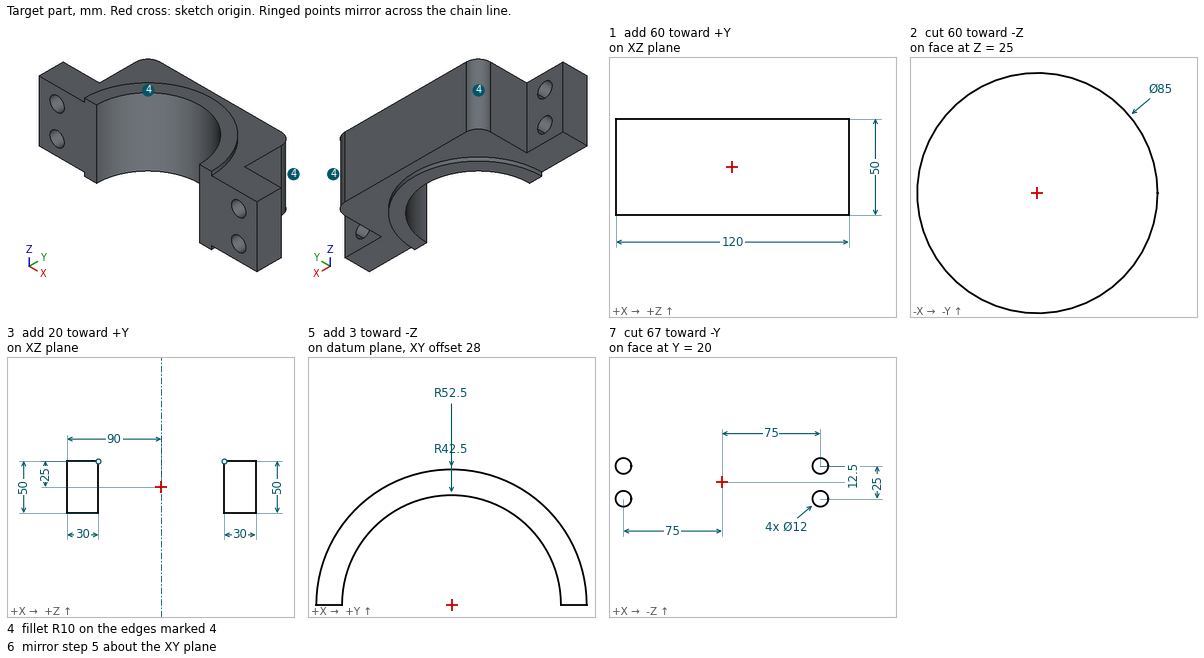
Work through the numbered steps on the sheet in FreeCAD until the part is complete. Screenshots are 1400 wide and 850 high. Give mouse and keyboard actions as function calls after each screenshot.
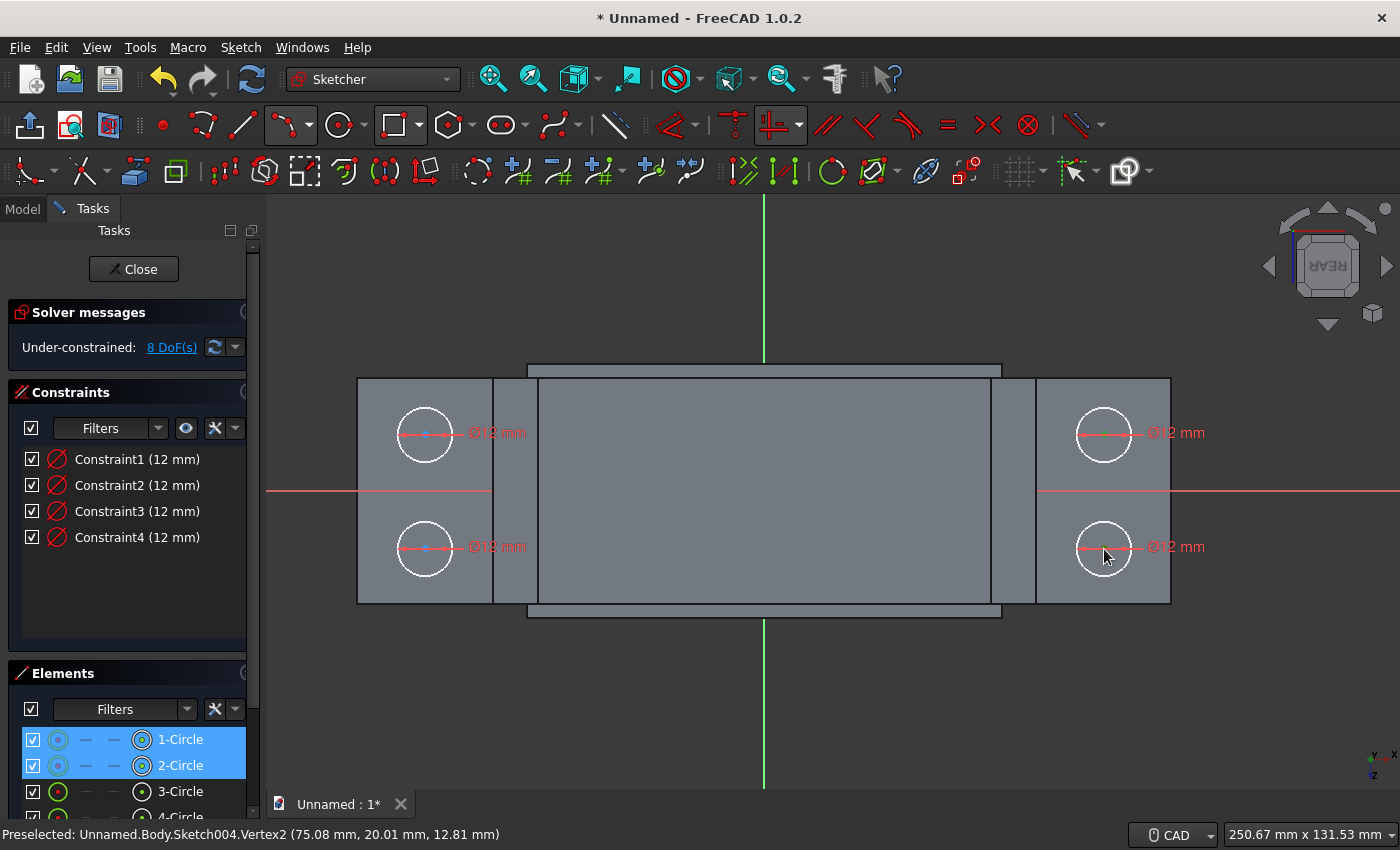
click(802, 126)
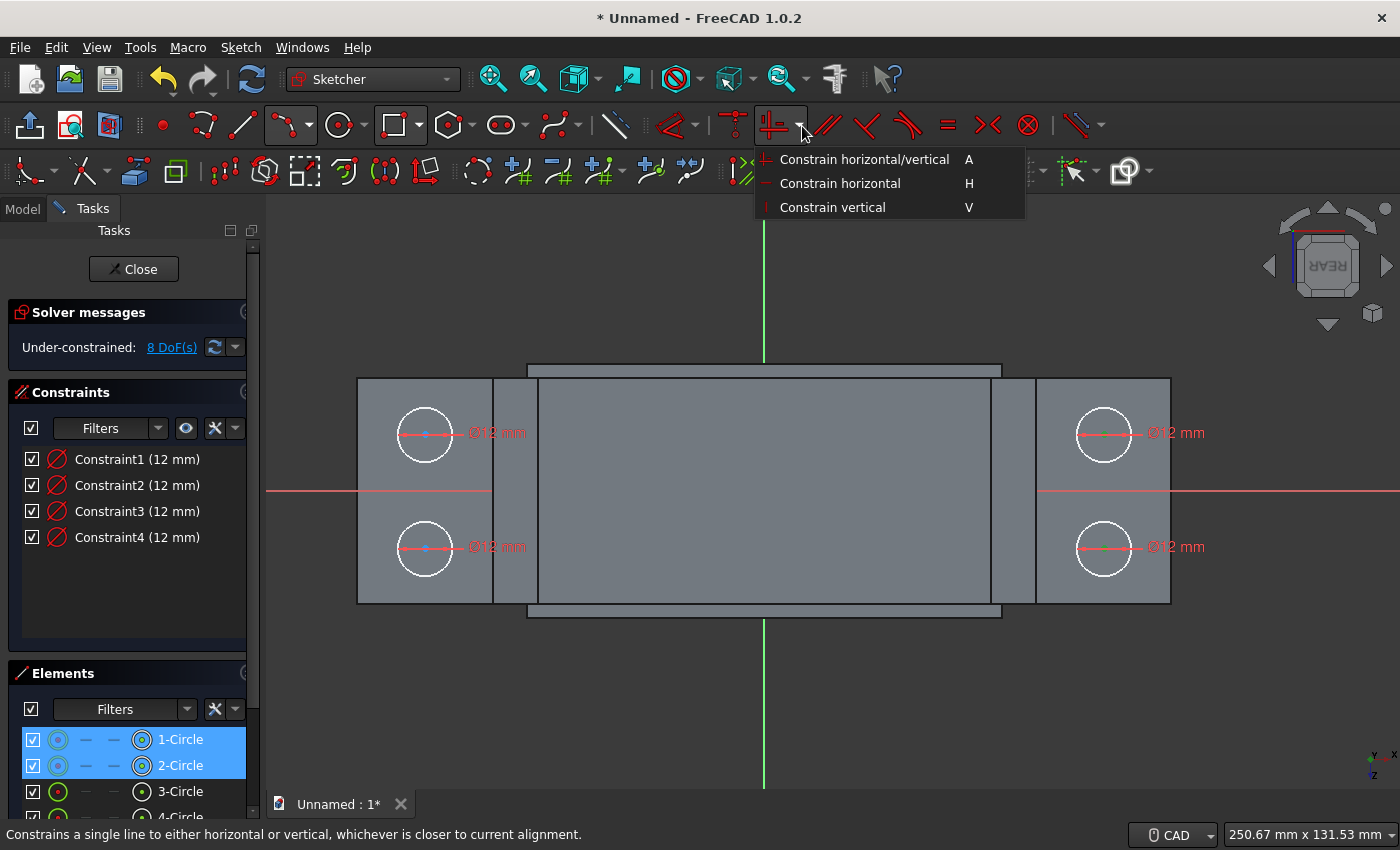
click(890, 207)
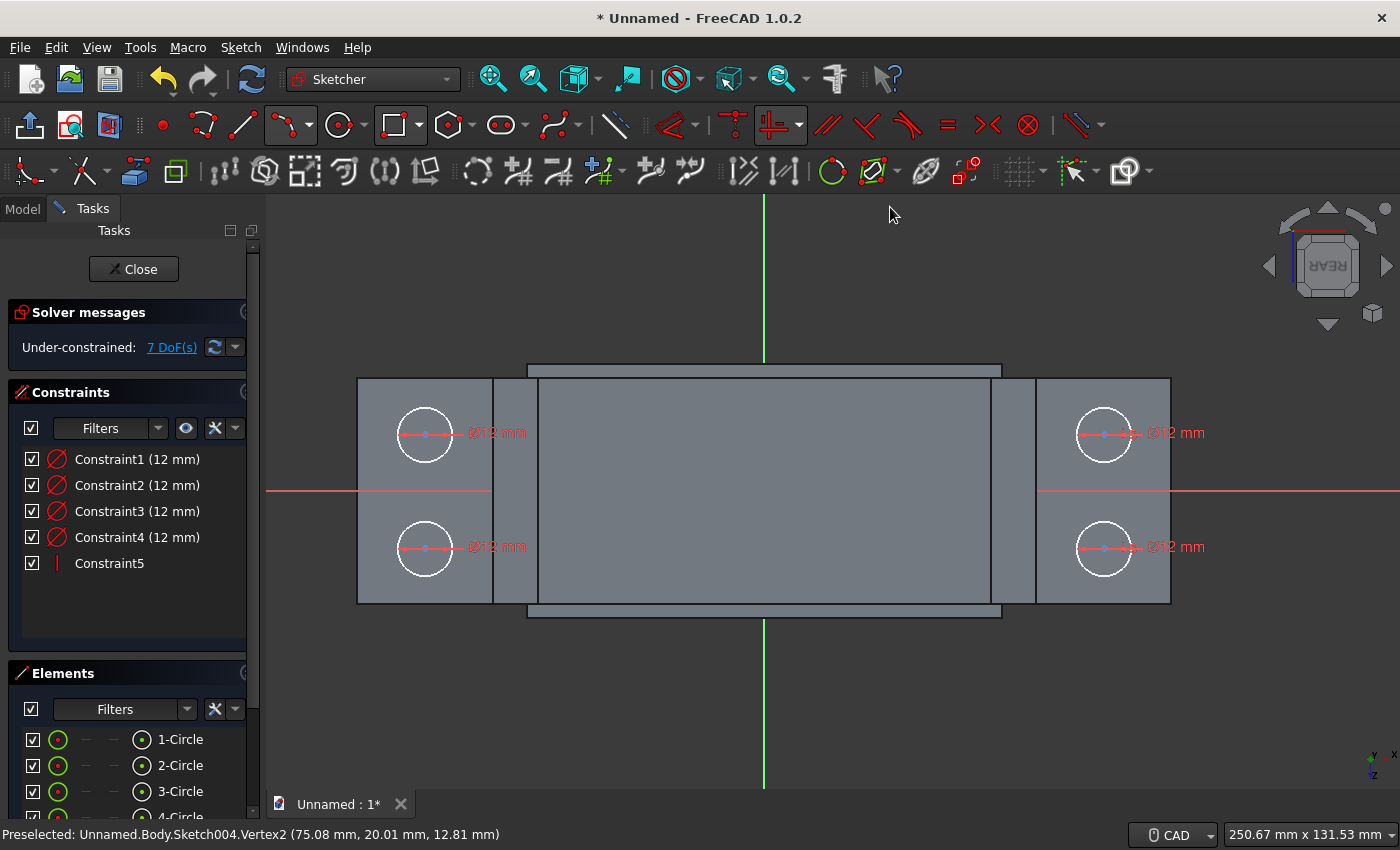
click(1104, 549)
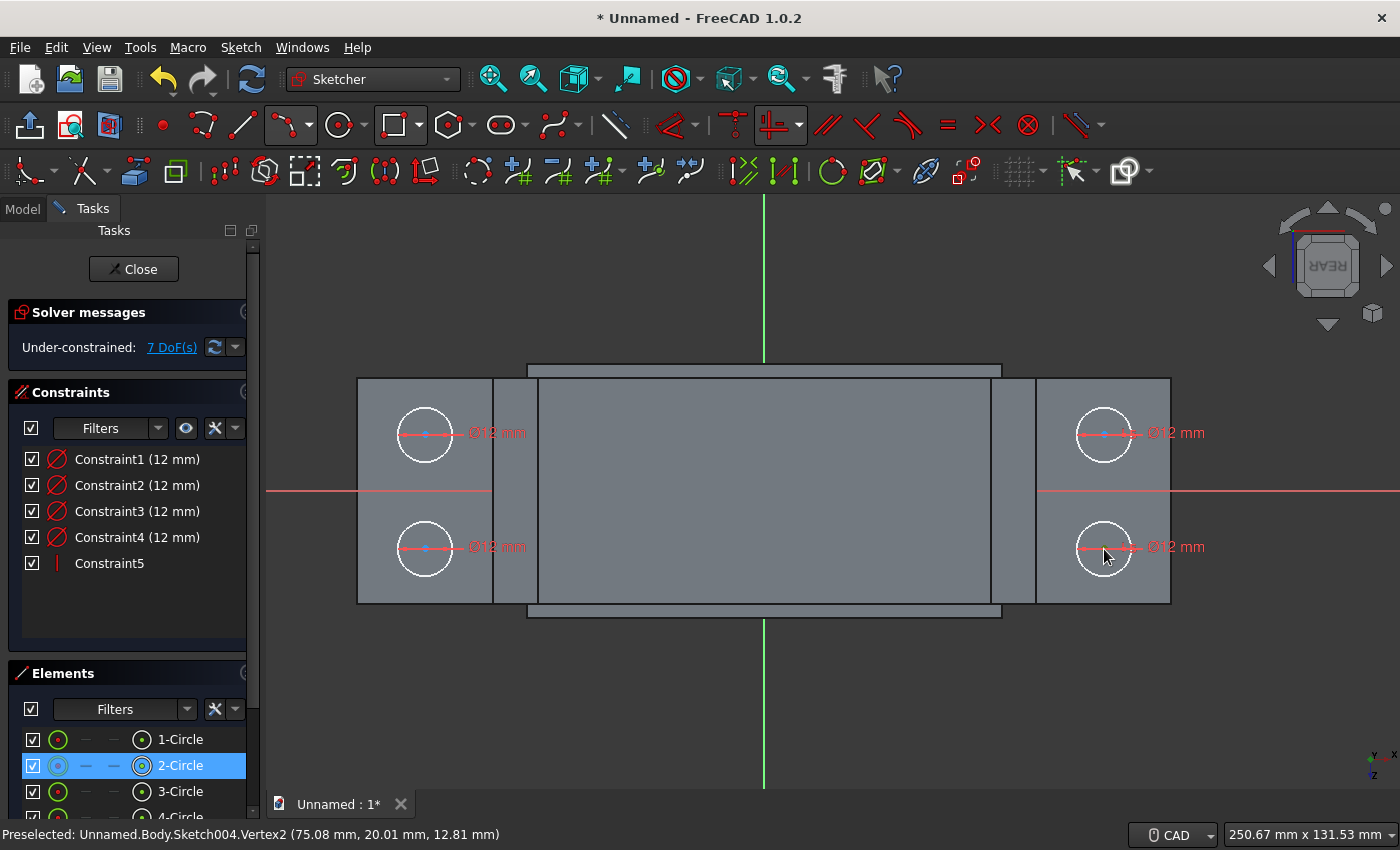
click(425, 549)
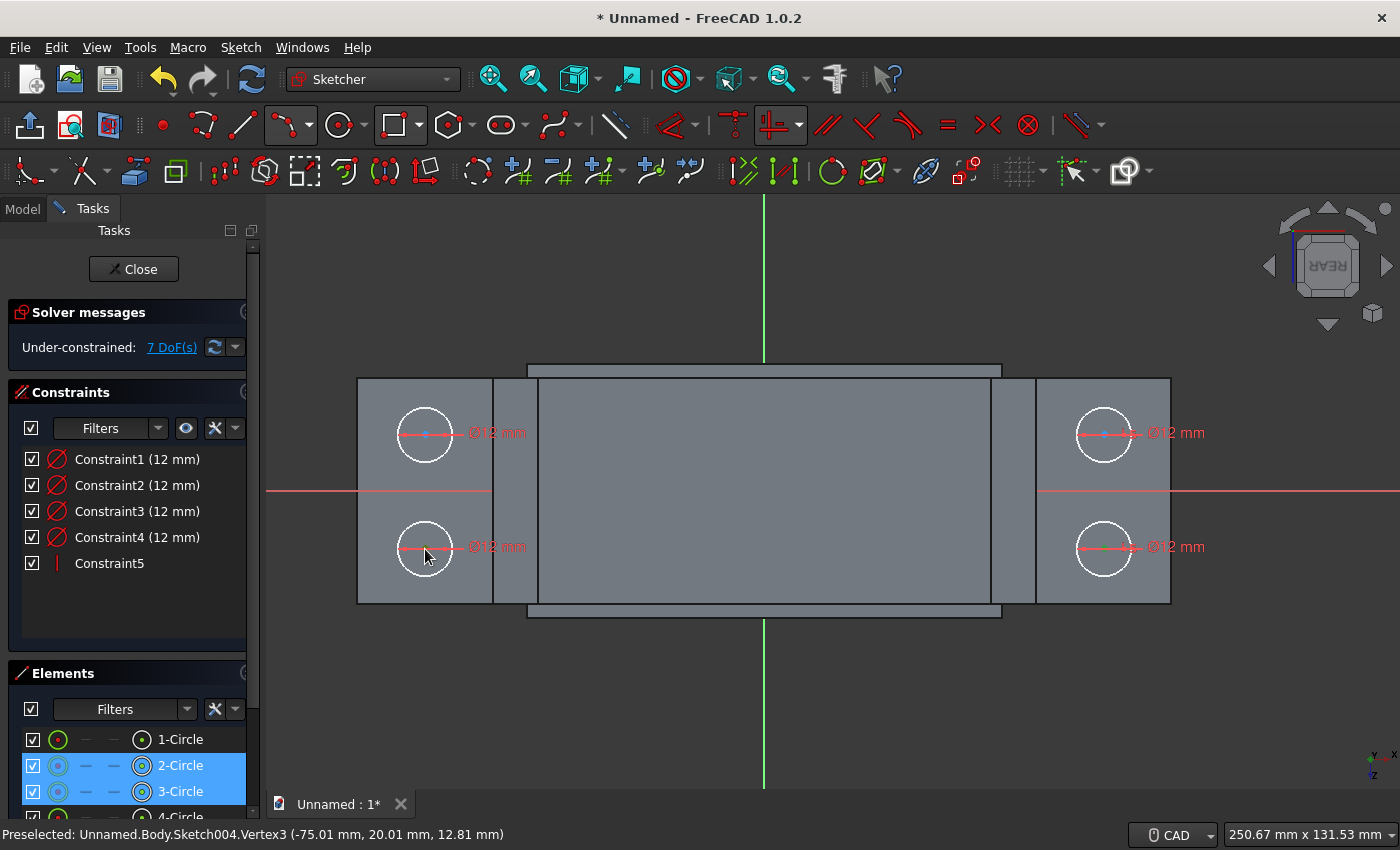
click(802, 126)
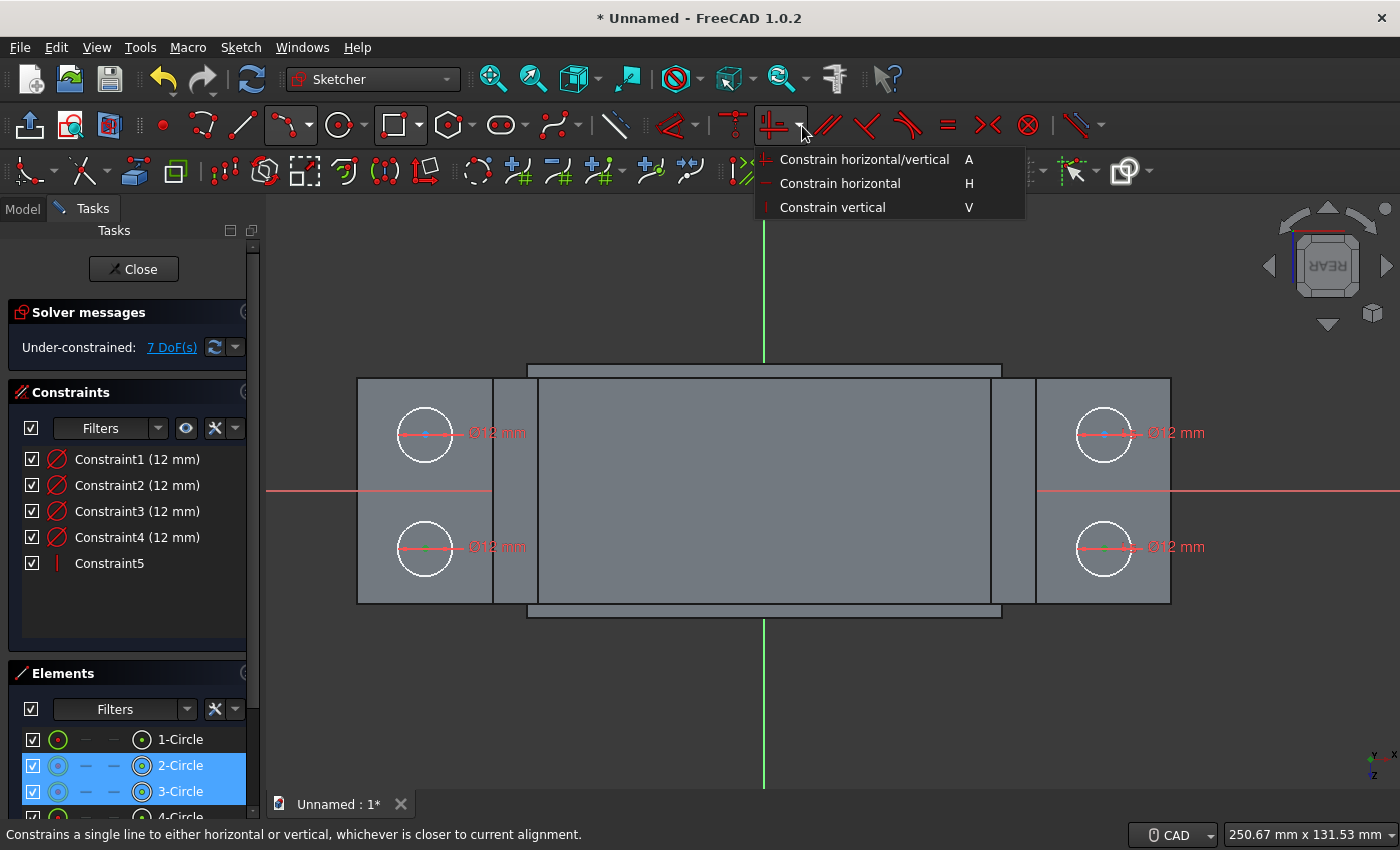
click(890, 183)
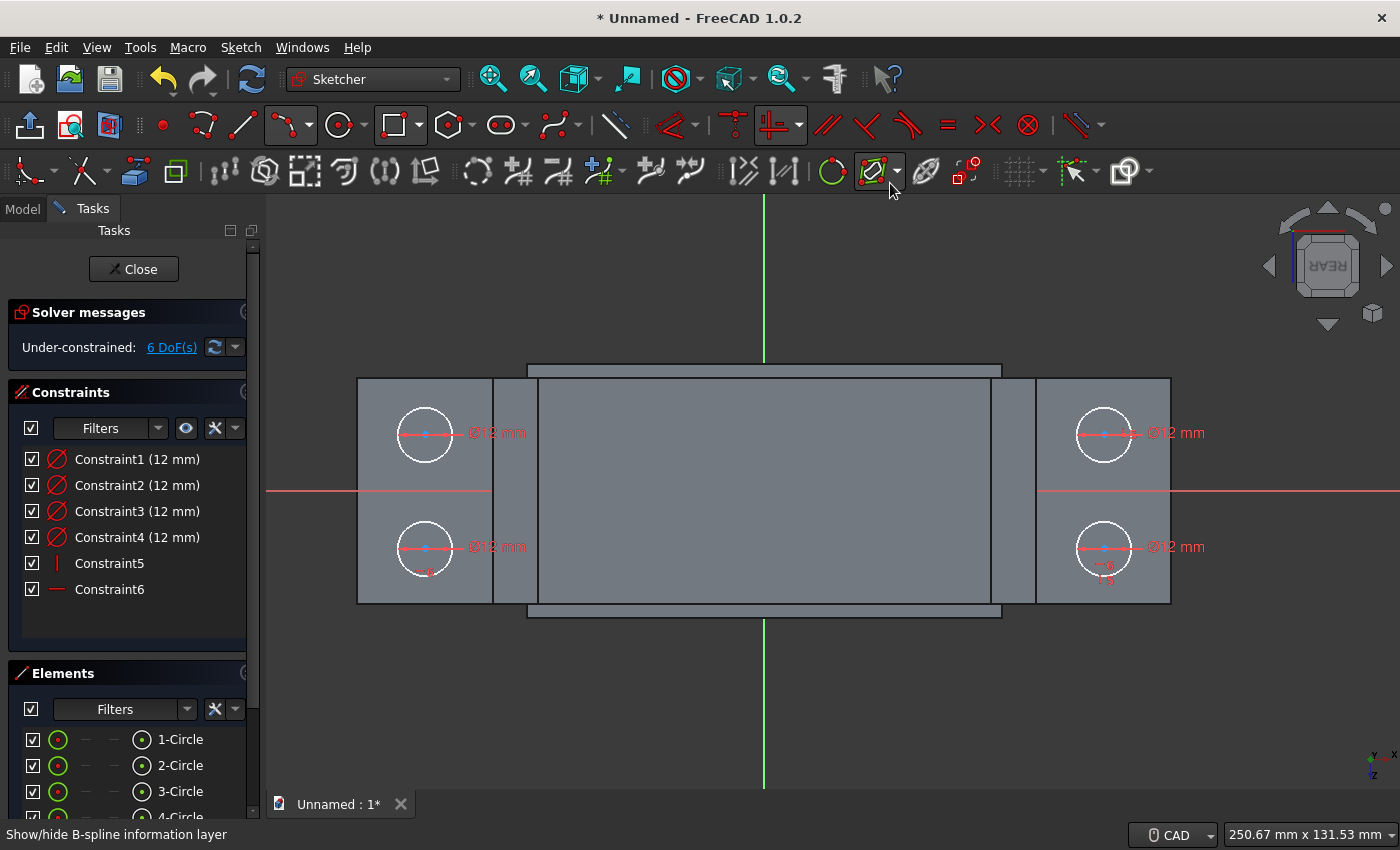
click(425, 549)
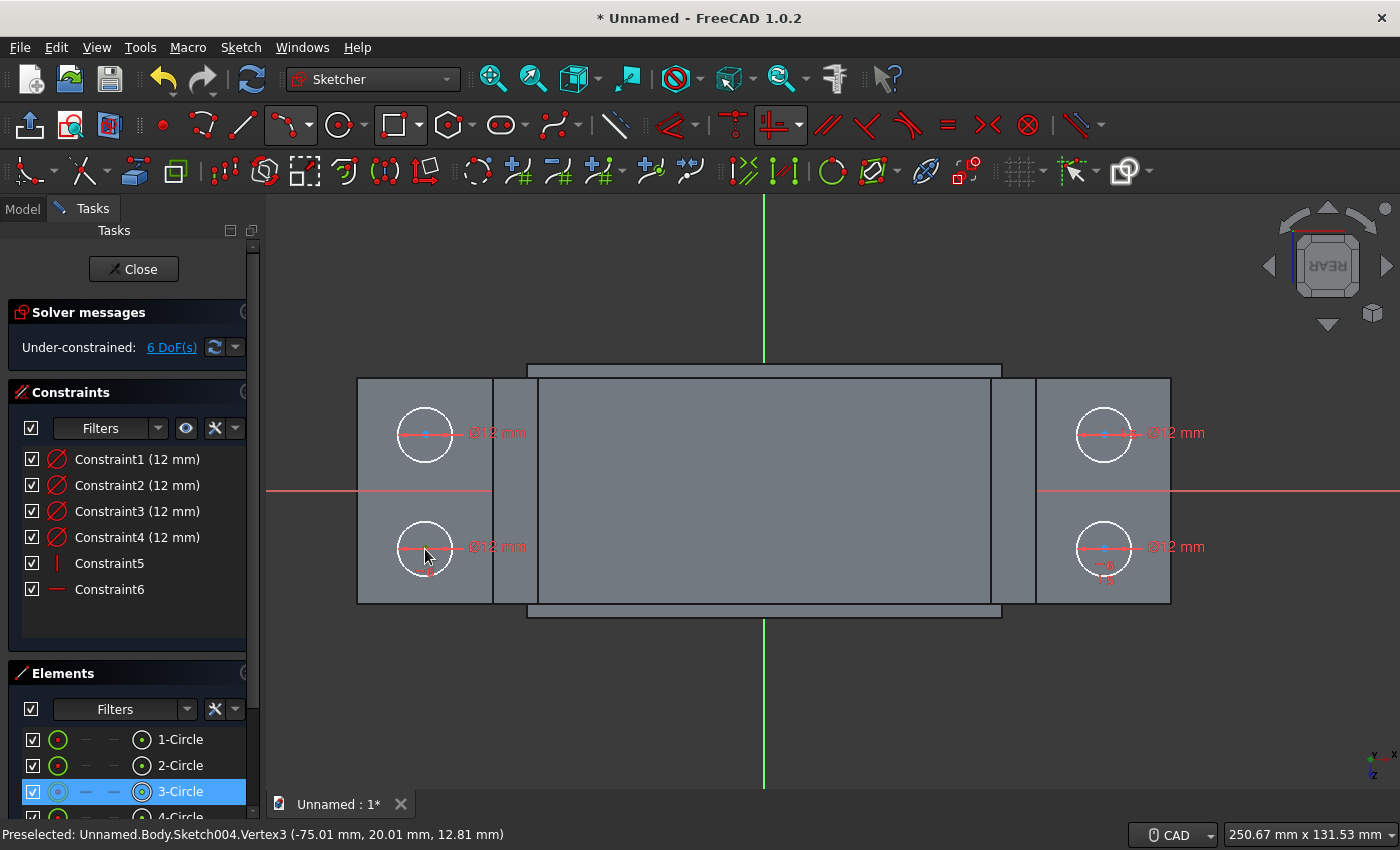
click(425, 435)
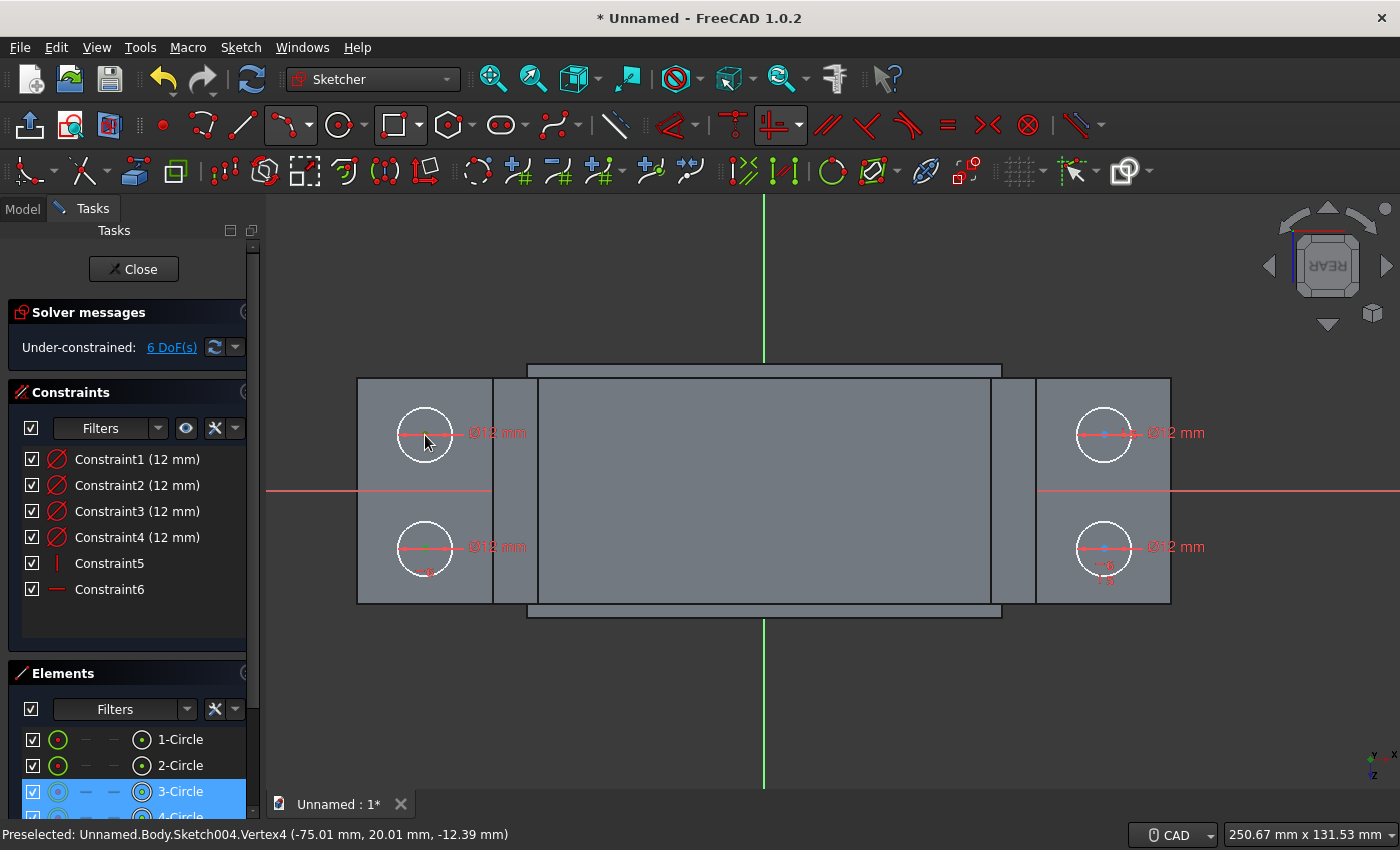
key(v)